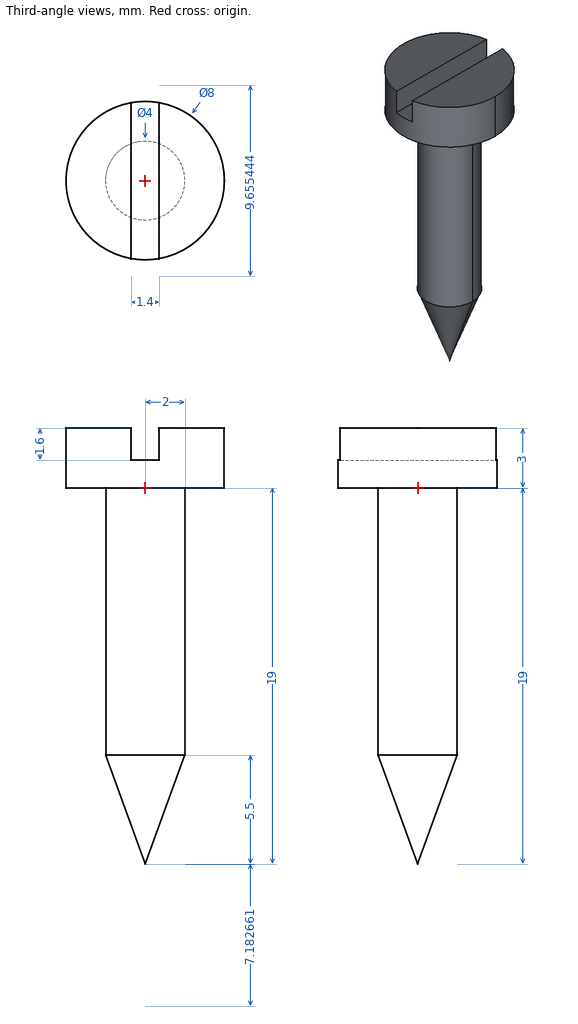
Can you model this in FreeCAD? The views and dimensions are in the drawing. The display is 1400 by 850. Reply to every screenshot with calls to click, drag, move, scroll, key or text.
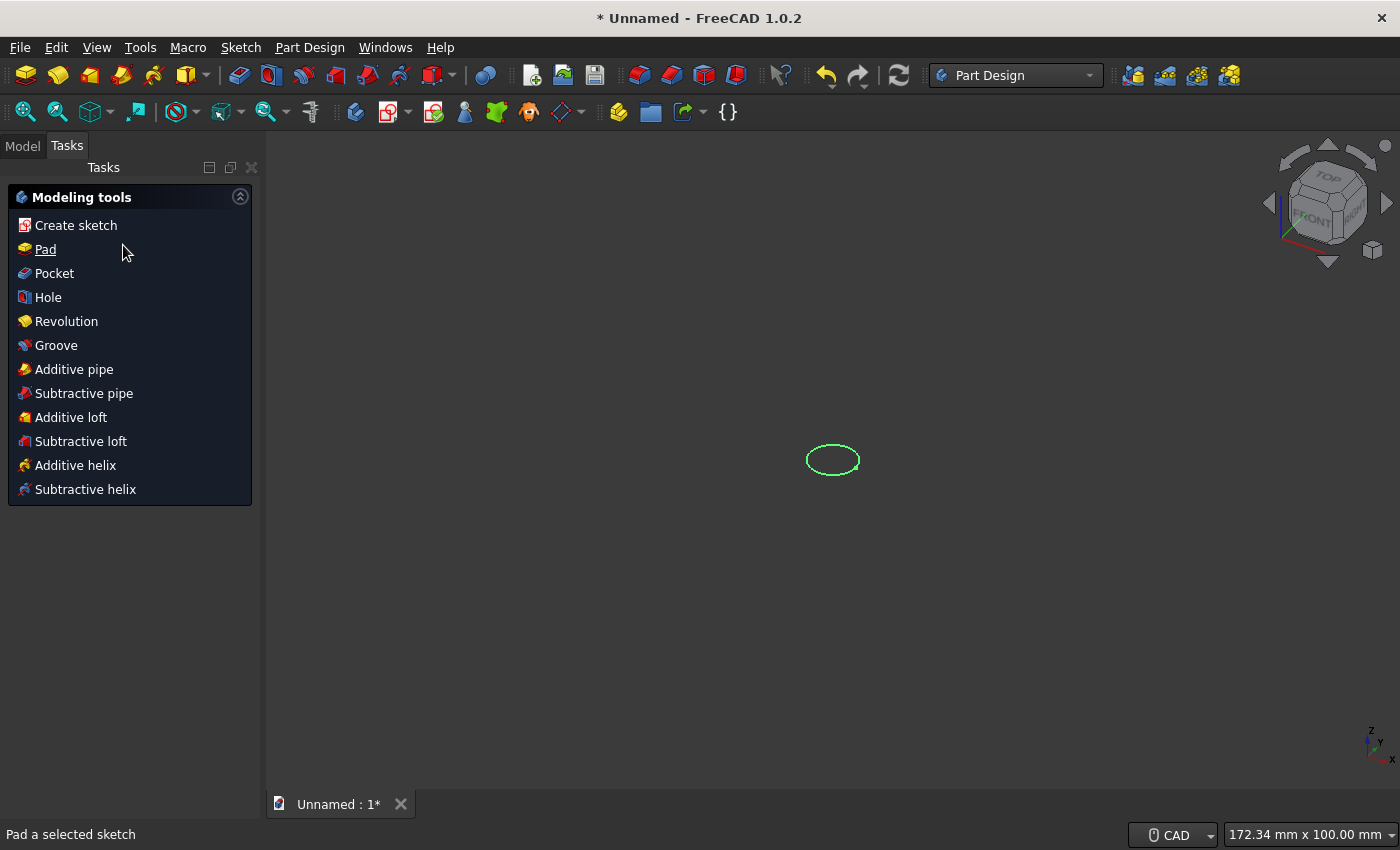
click(26, 76)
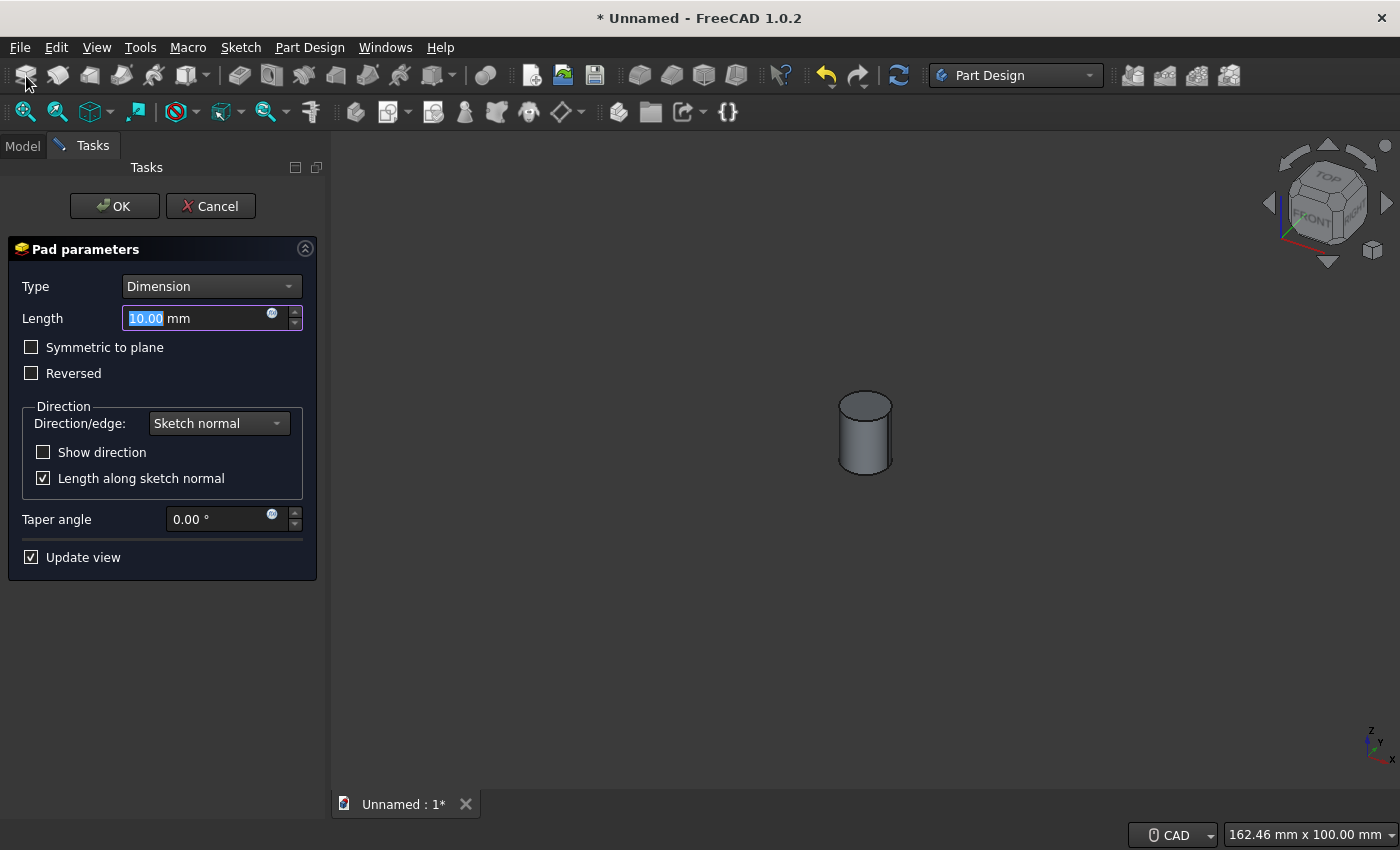
text(3)
key(Tab)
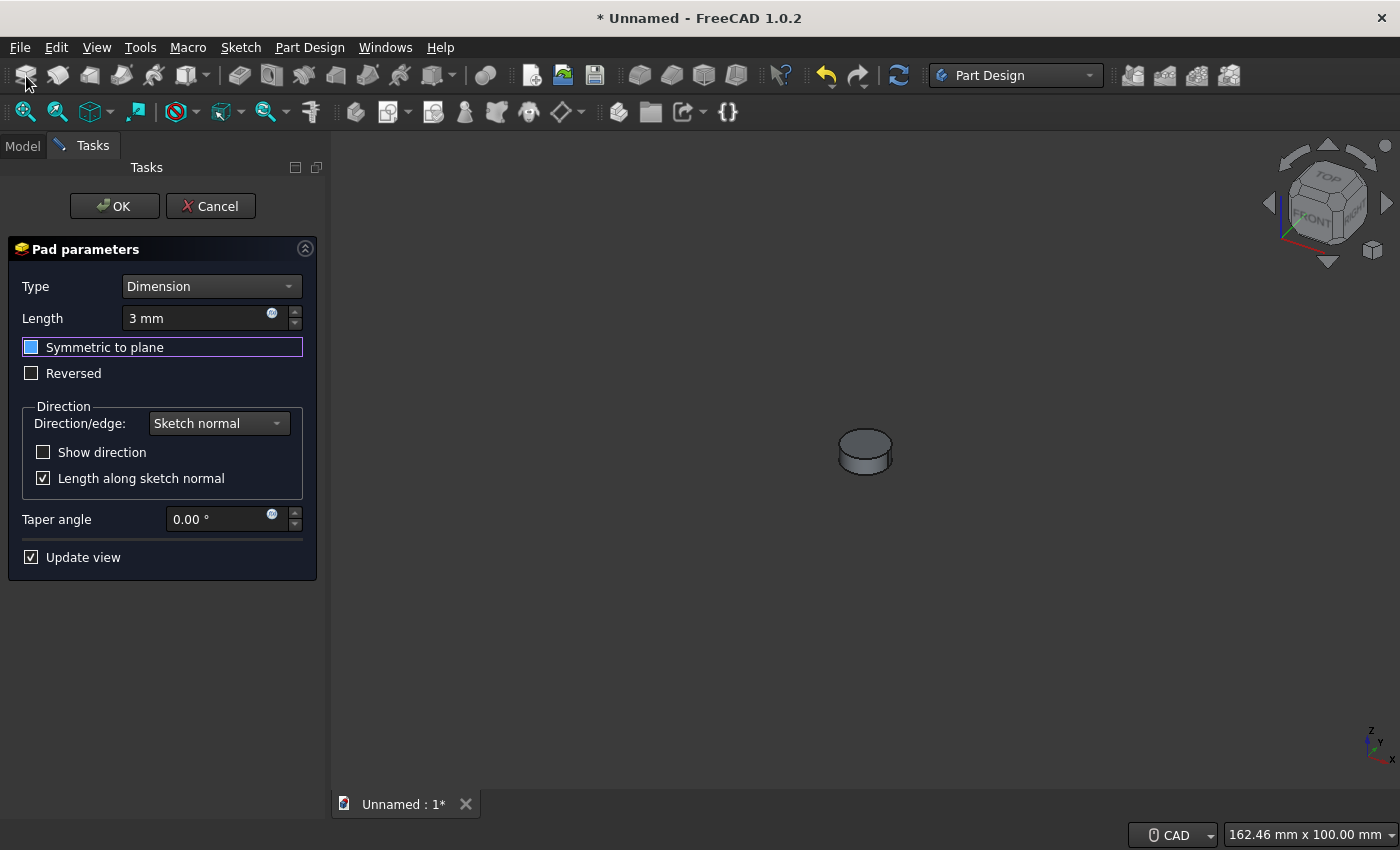
click(115, 206)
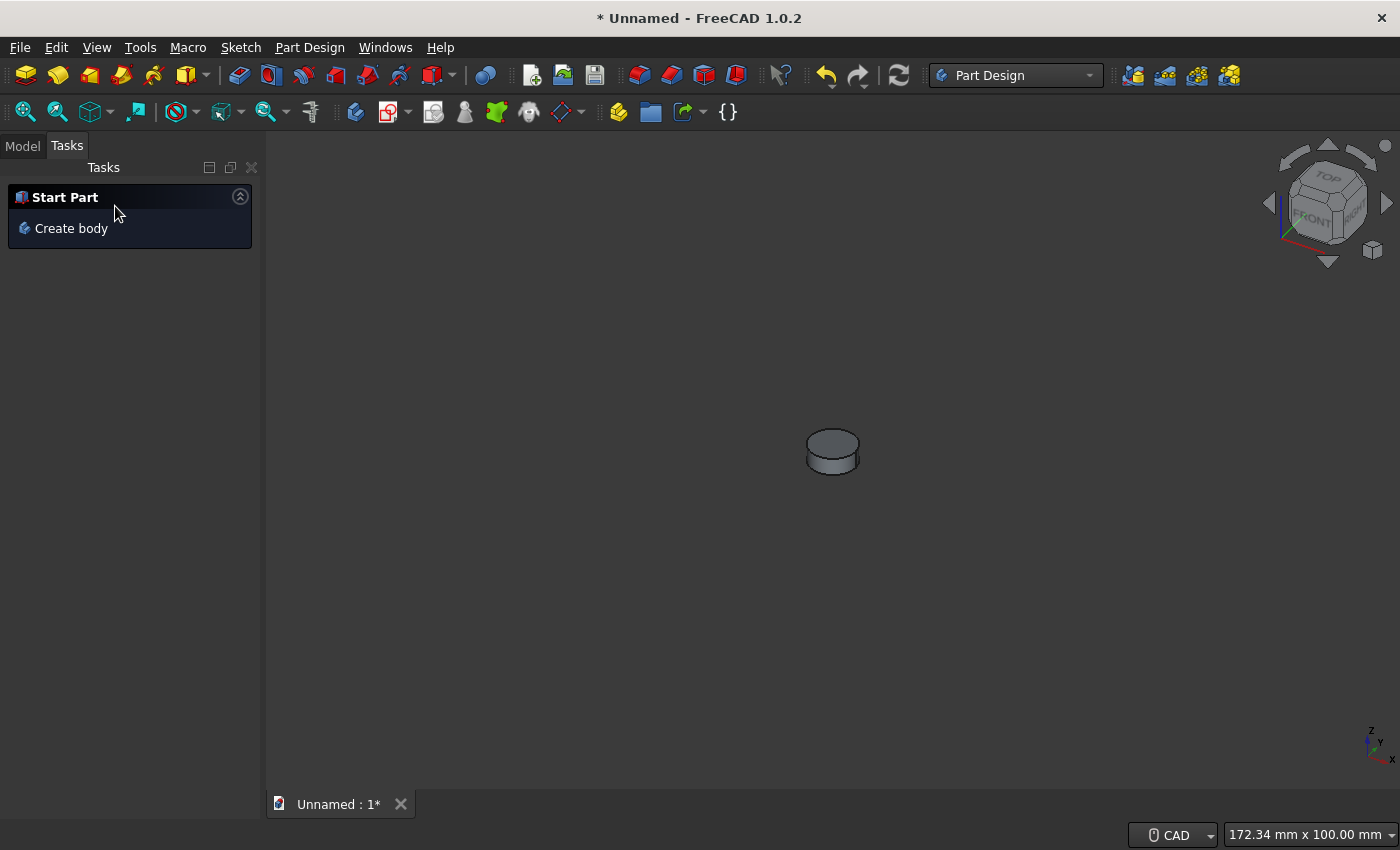
click(26, 112)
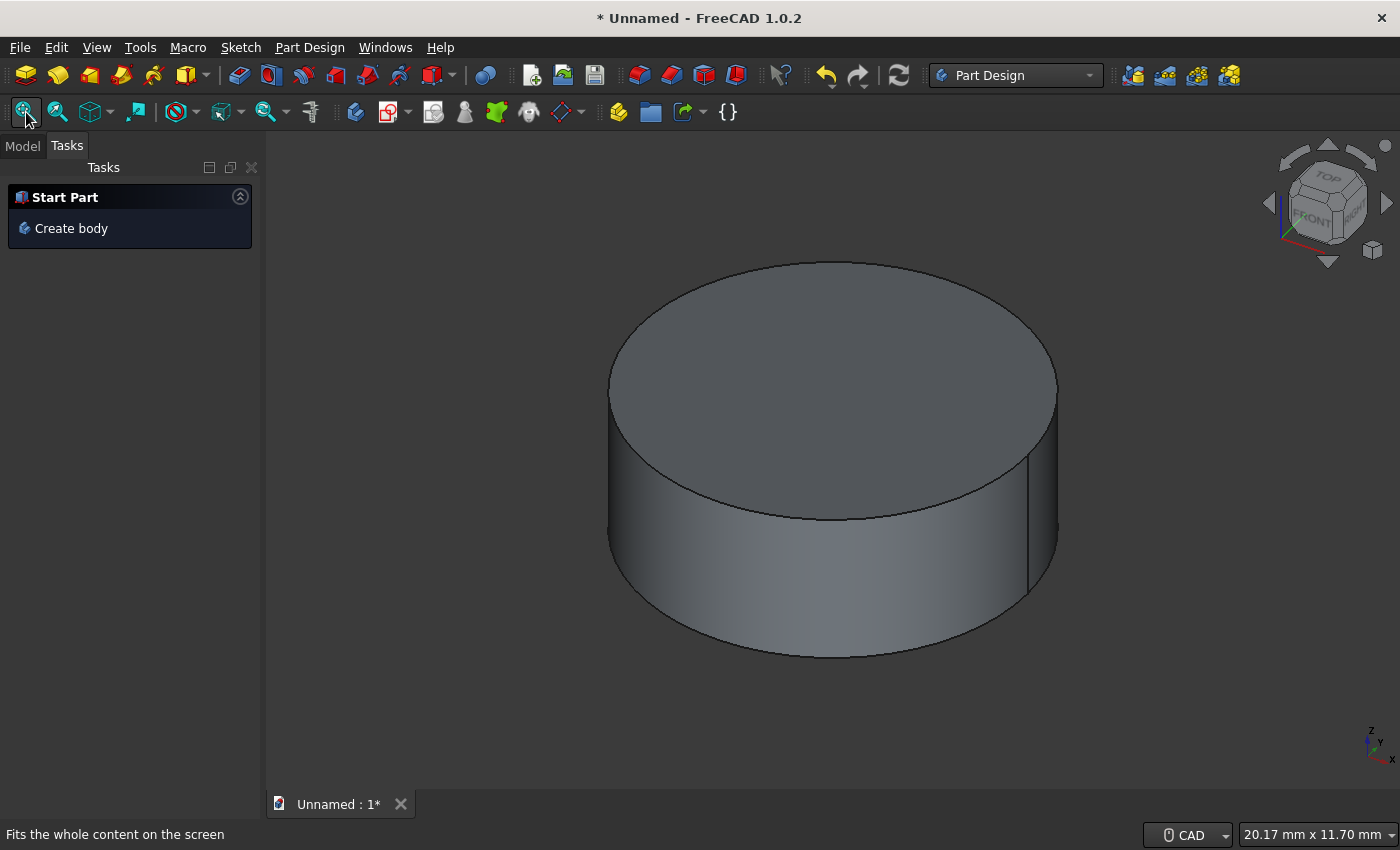
click(833, 390)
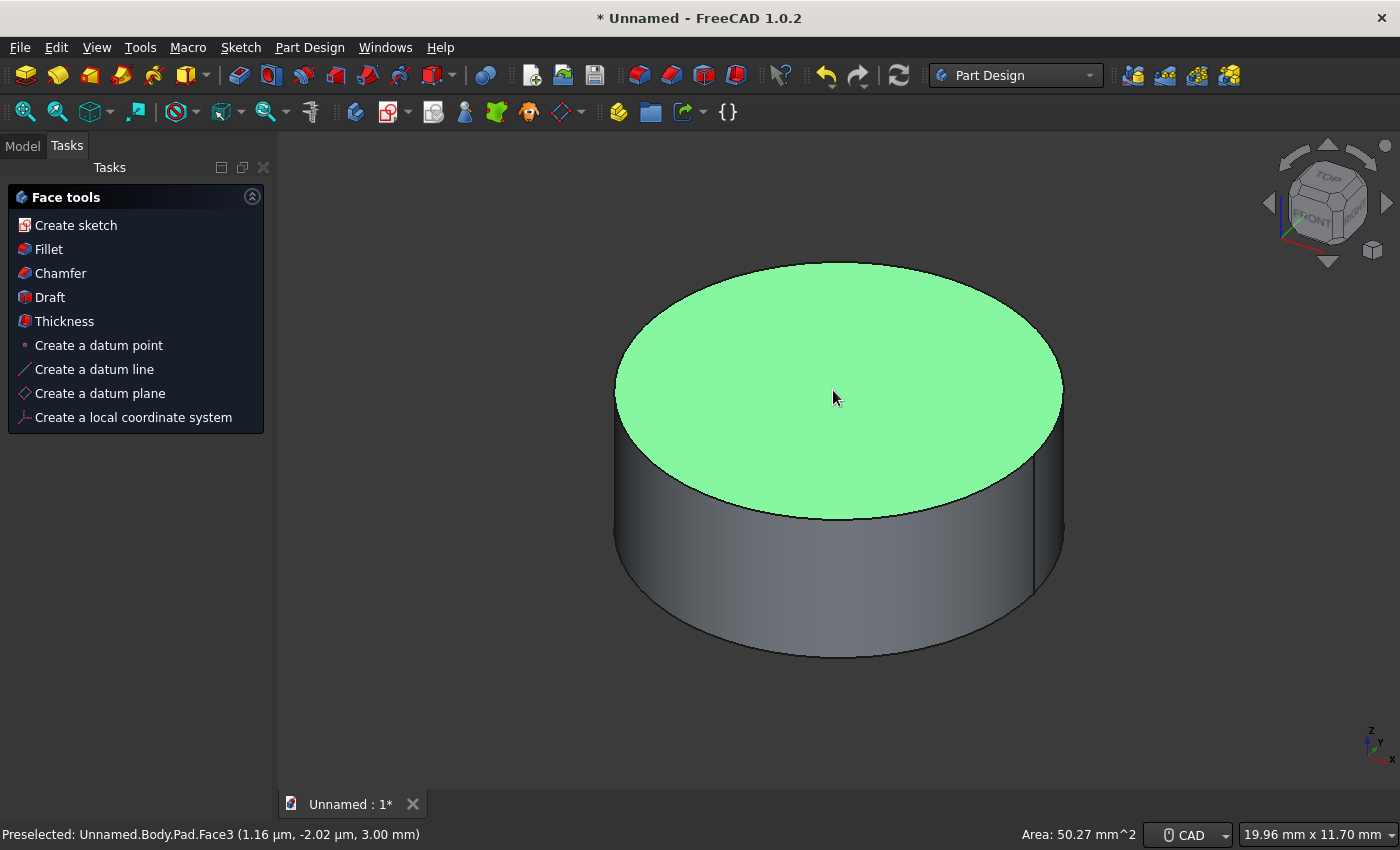
click(388, 112)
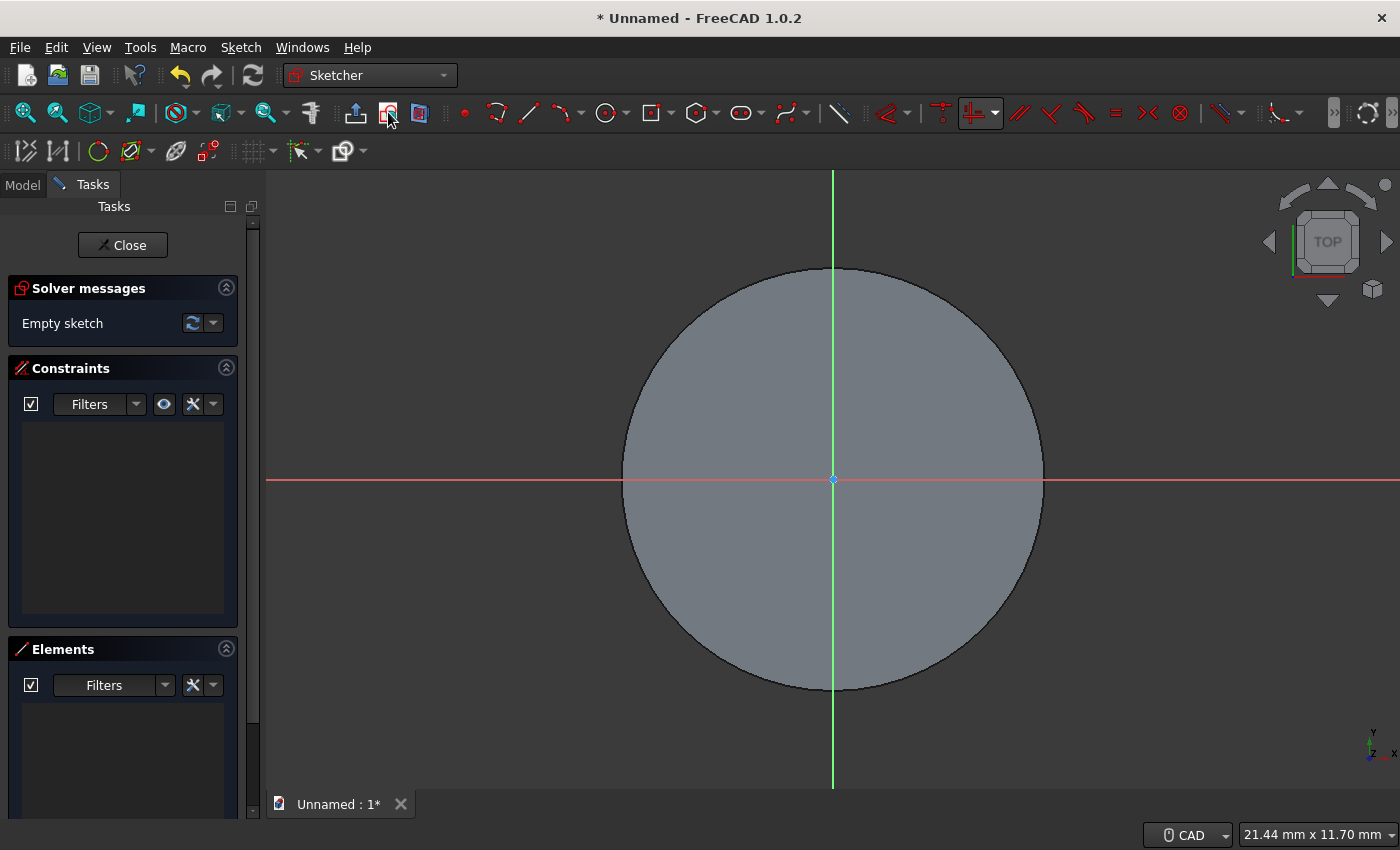
key(g)
key(v)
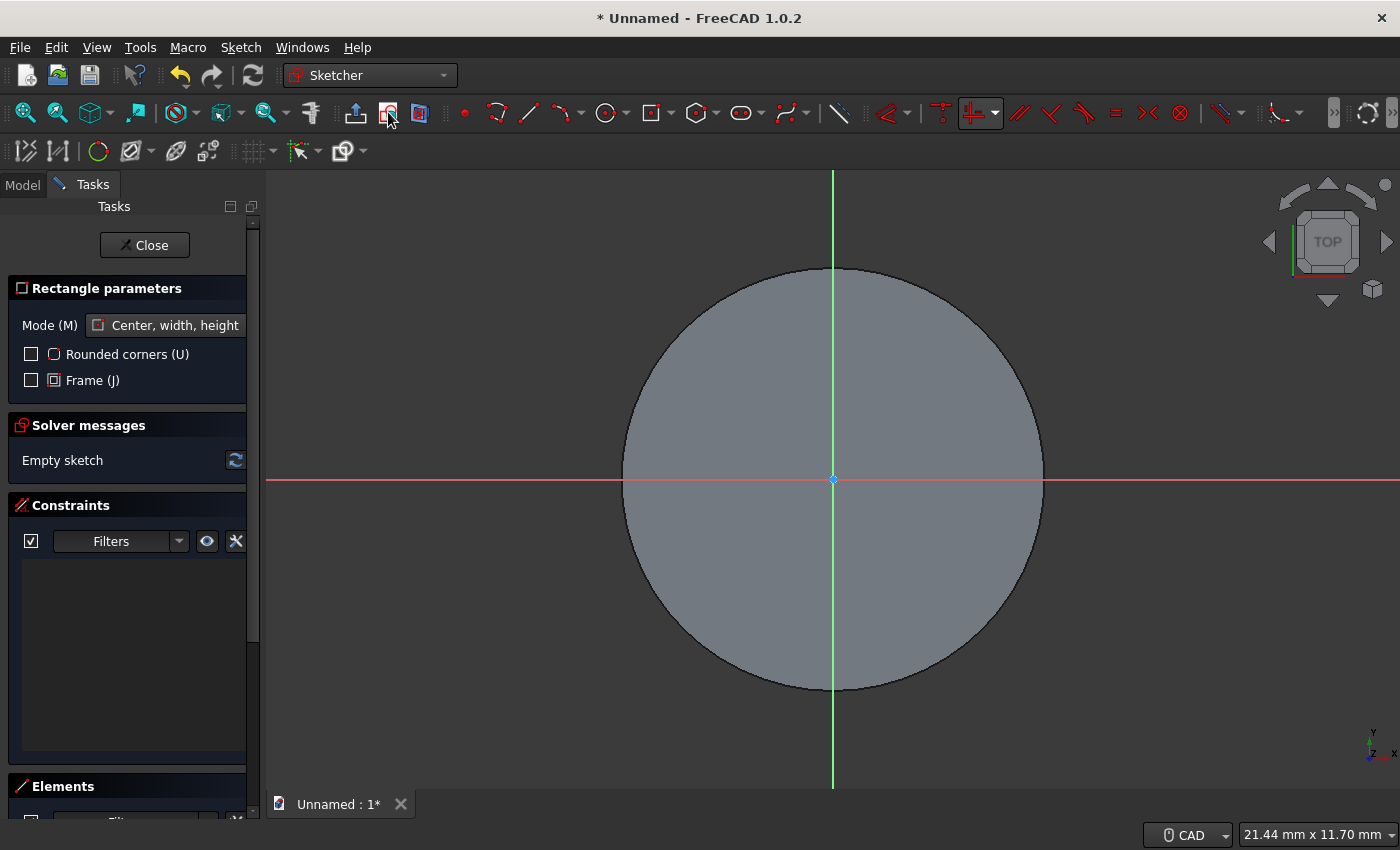
click(833, 480)
move(870, 224)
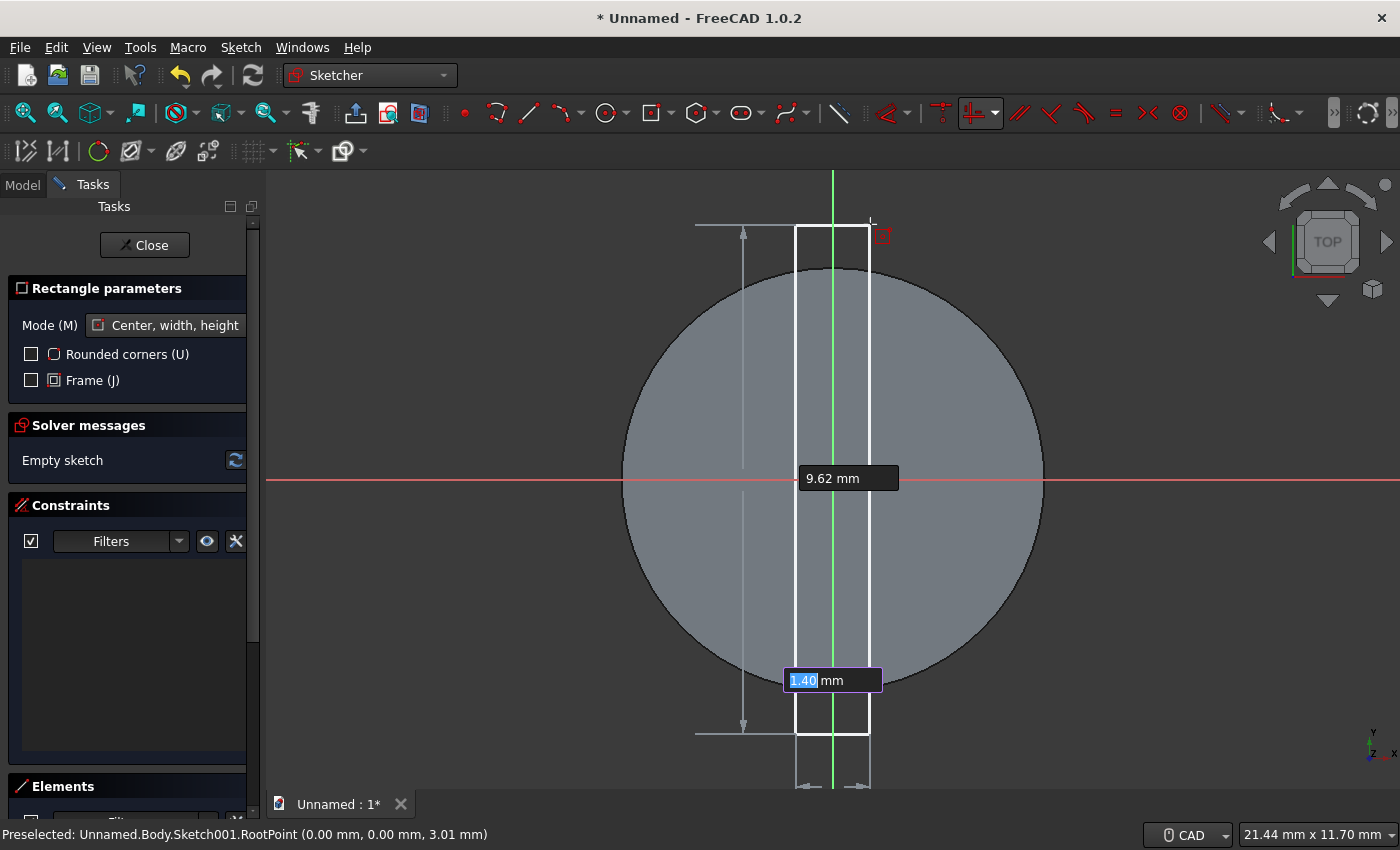
text(1.4)
key(Tab)
text(9.655444)
key(Return)
key(Escape)